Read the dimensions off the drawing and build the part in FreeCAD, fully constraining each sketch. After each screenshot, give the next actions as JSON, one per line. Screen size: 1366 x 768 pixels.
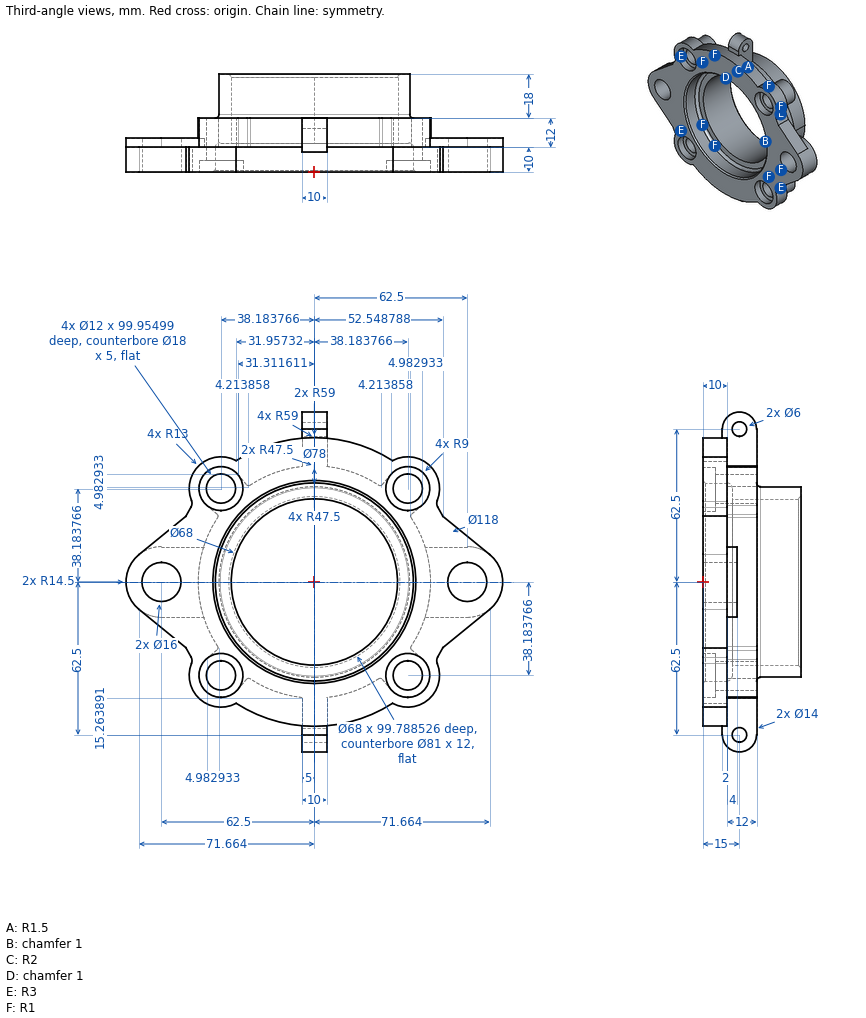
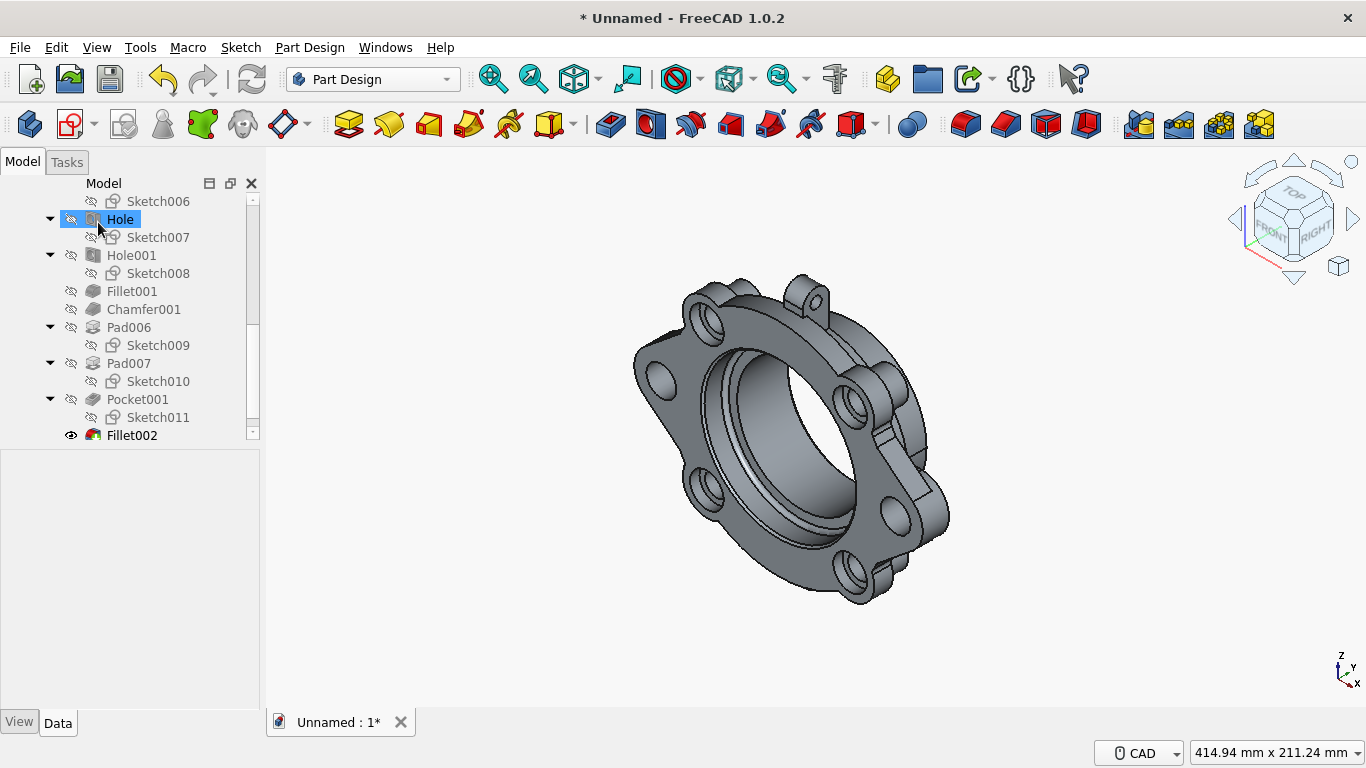
{"action": "key", "text": "2"}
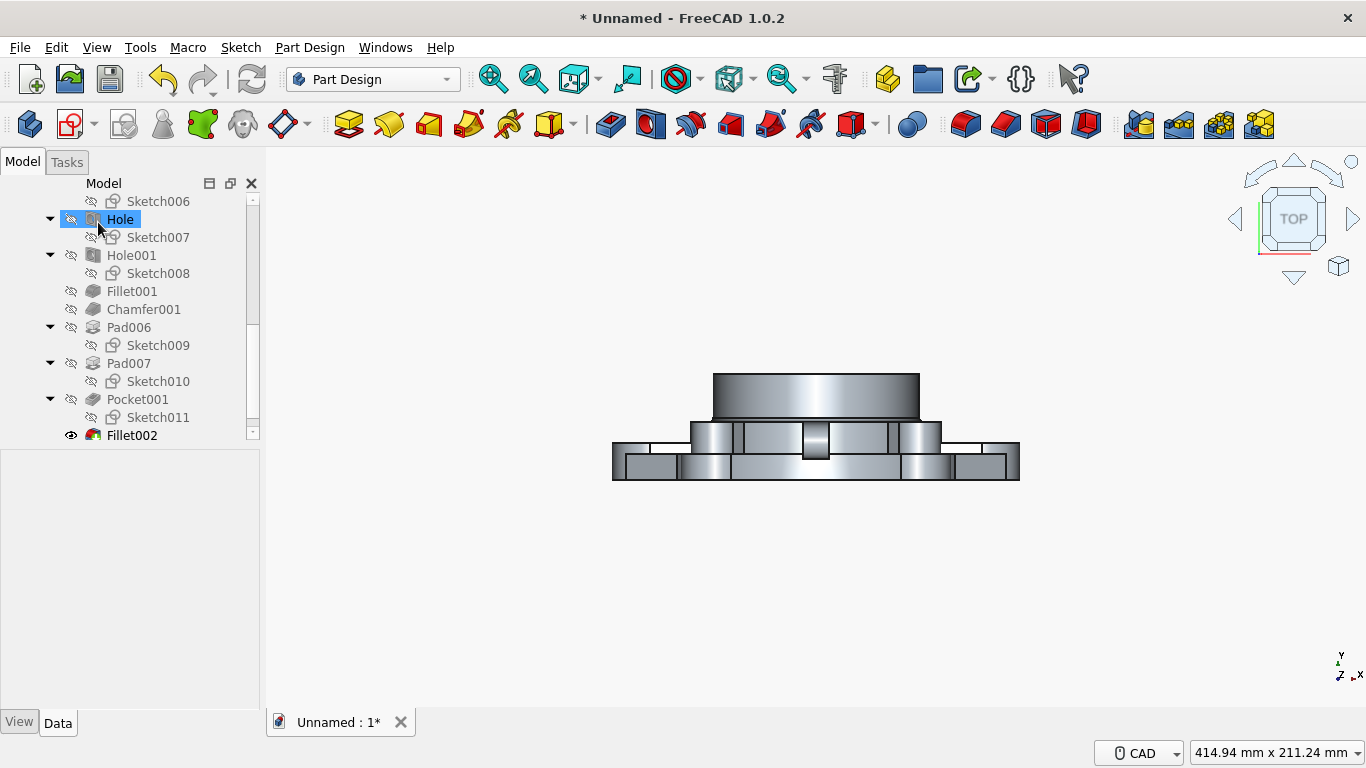
{"action": "left_click", "coordinate": [494, 80]}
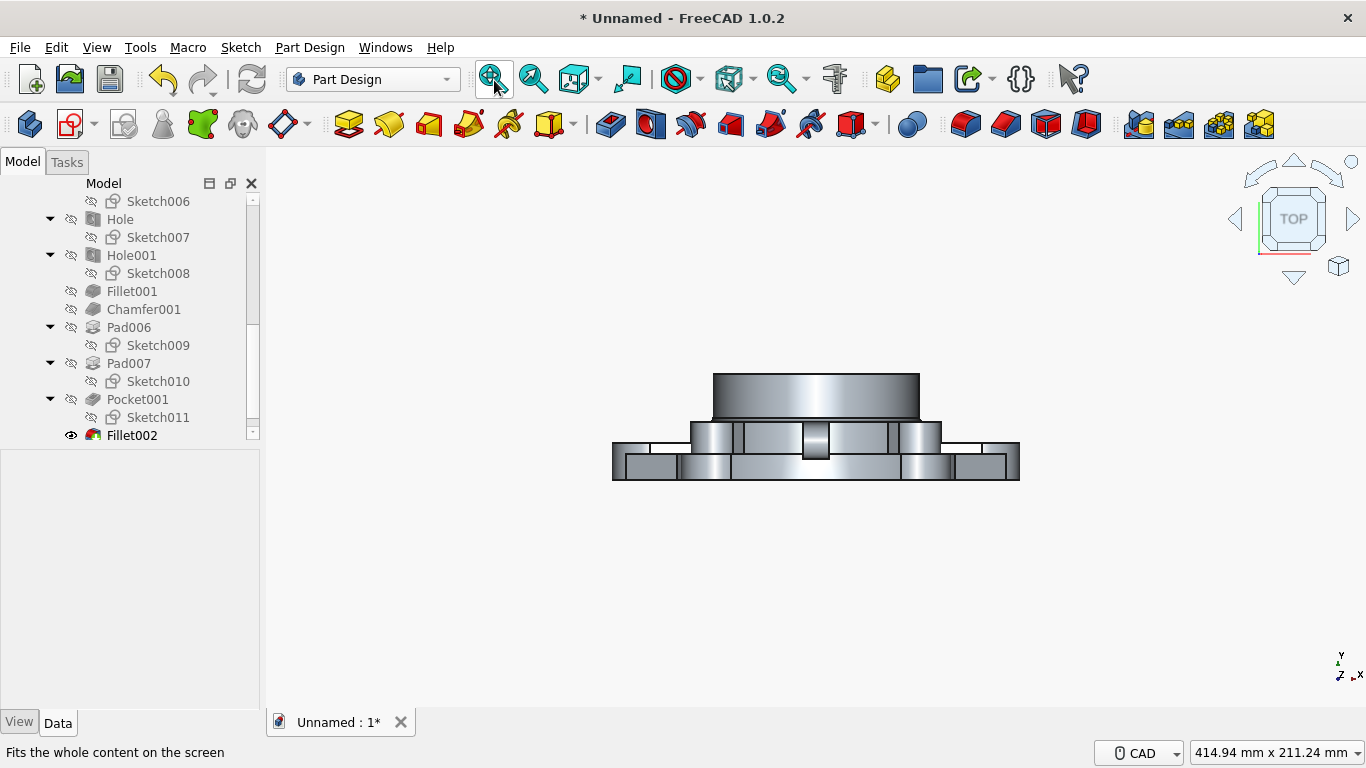
{"action": "key", "text": "1"}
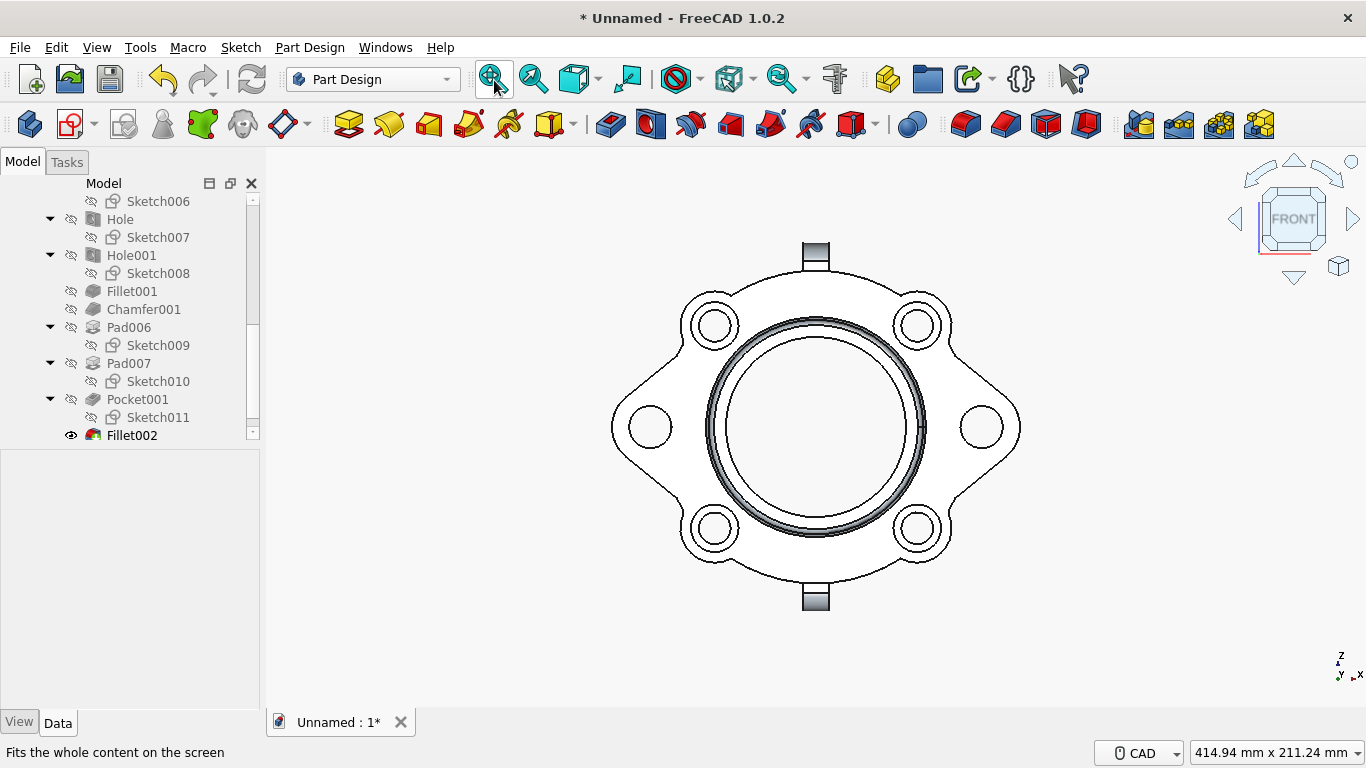
{"action": "key", "text": "3"}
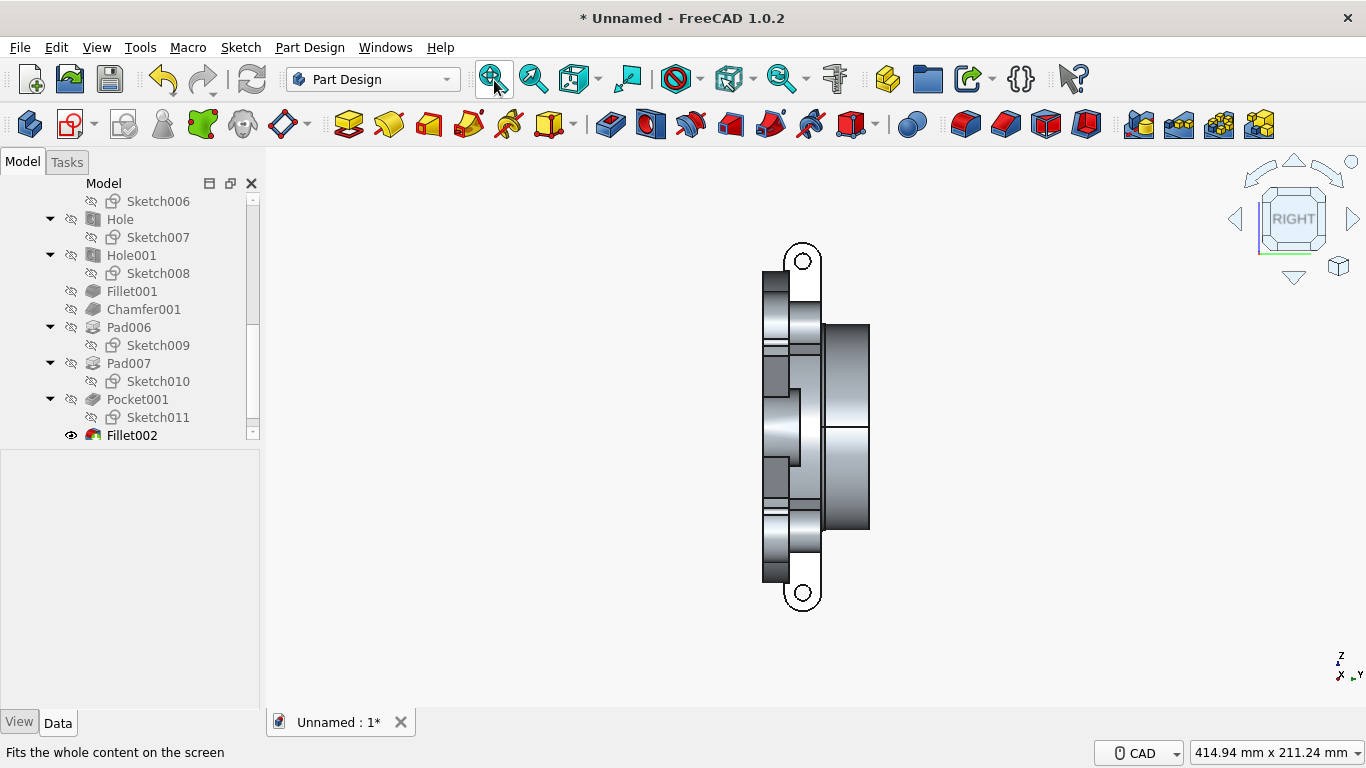
{"action": "key", "text": "5"}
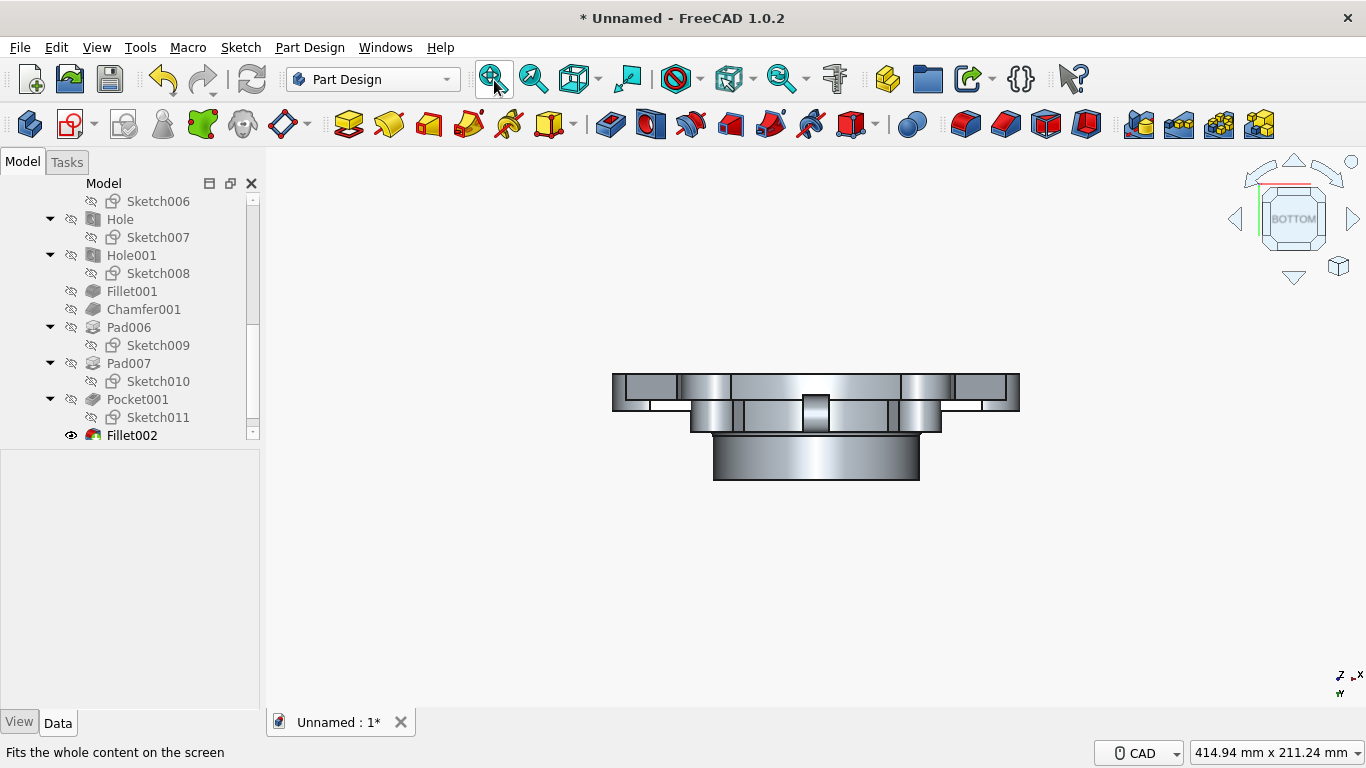
{"action": "left_click", "coordinate": [494, 80]}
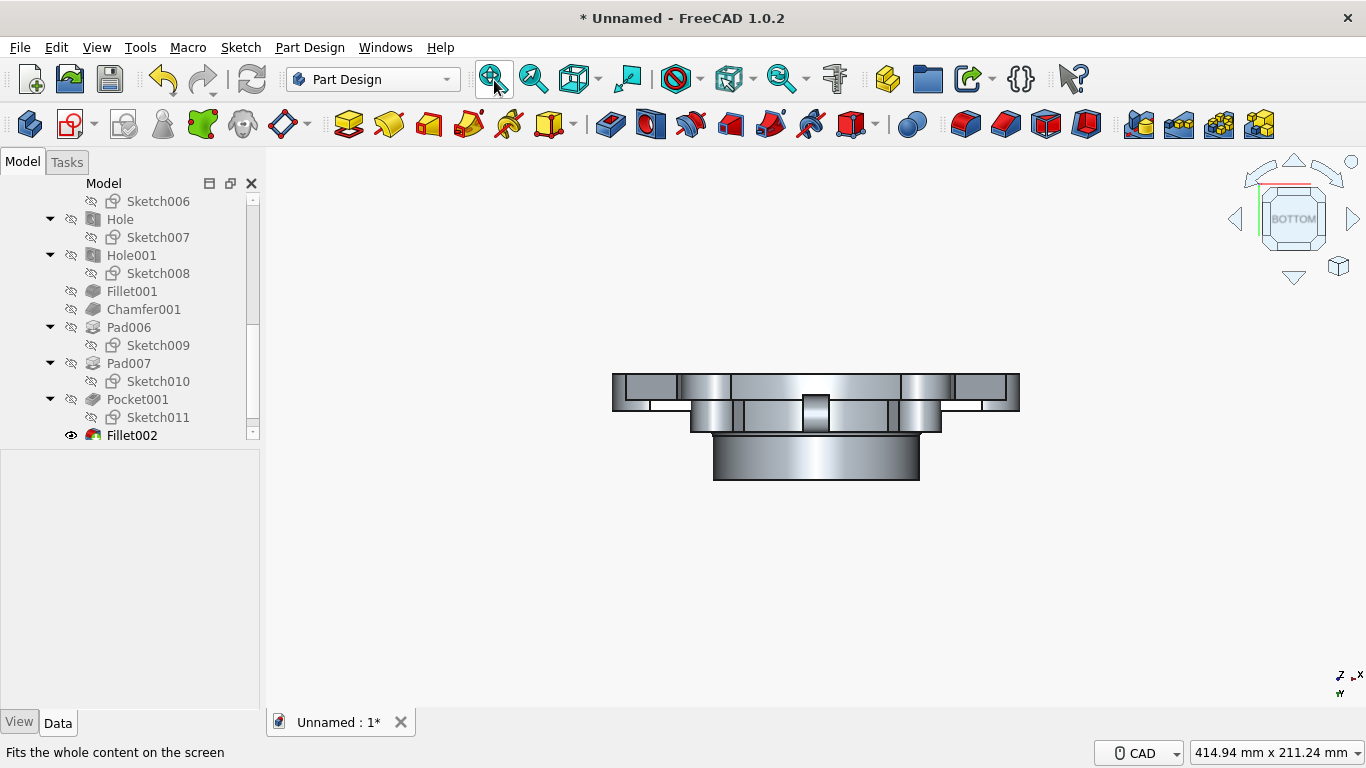
{"action": "key", "text": "4"}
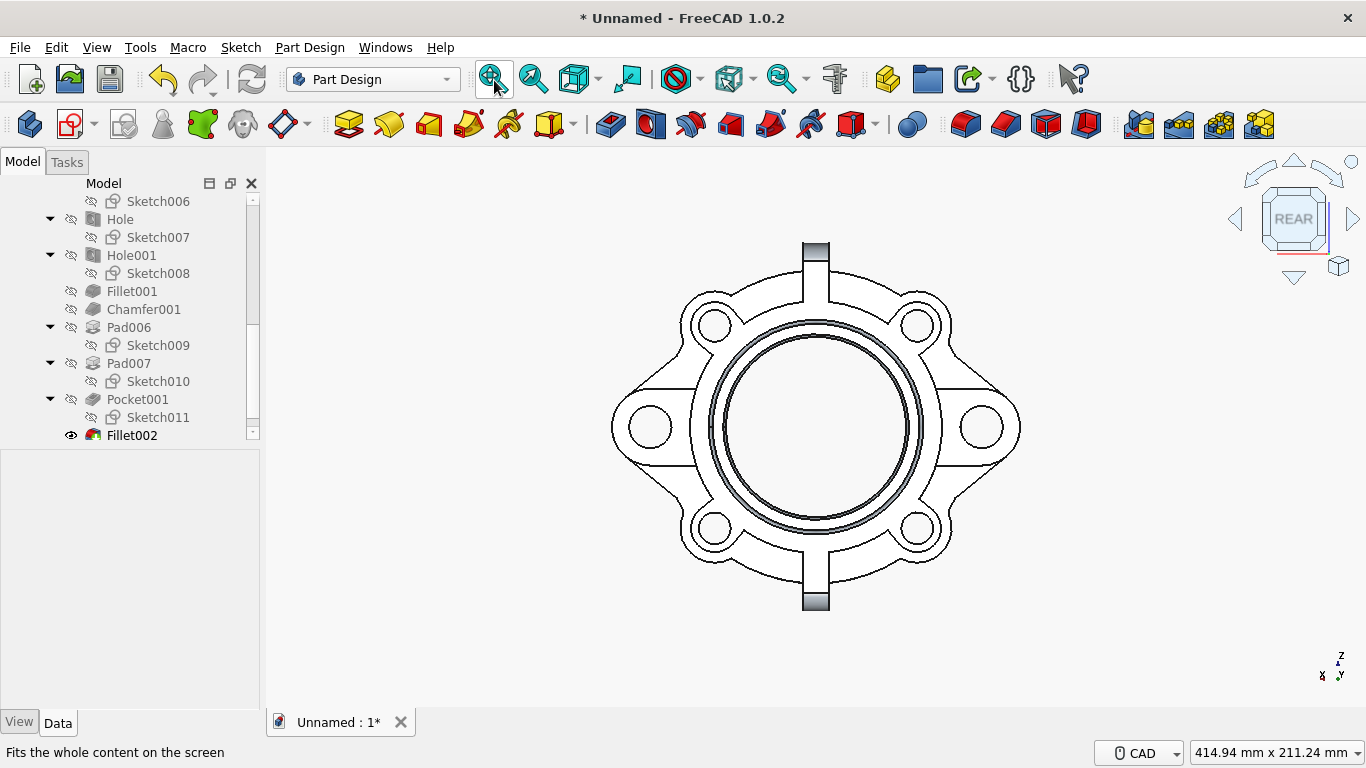
{"action": "key", "text": "6"}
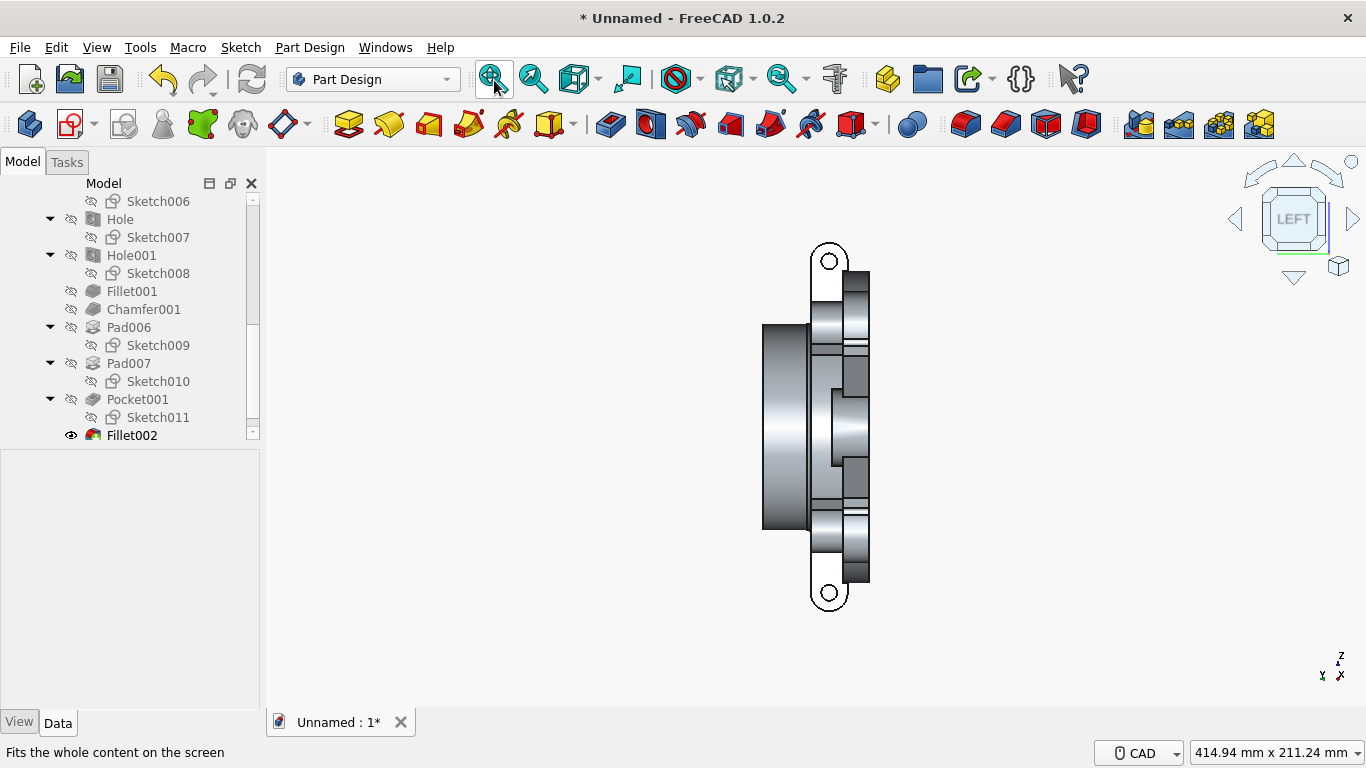
{"action": "key", "text": "v 3"}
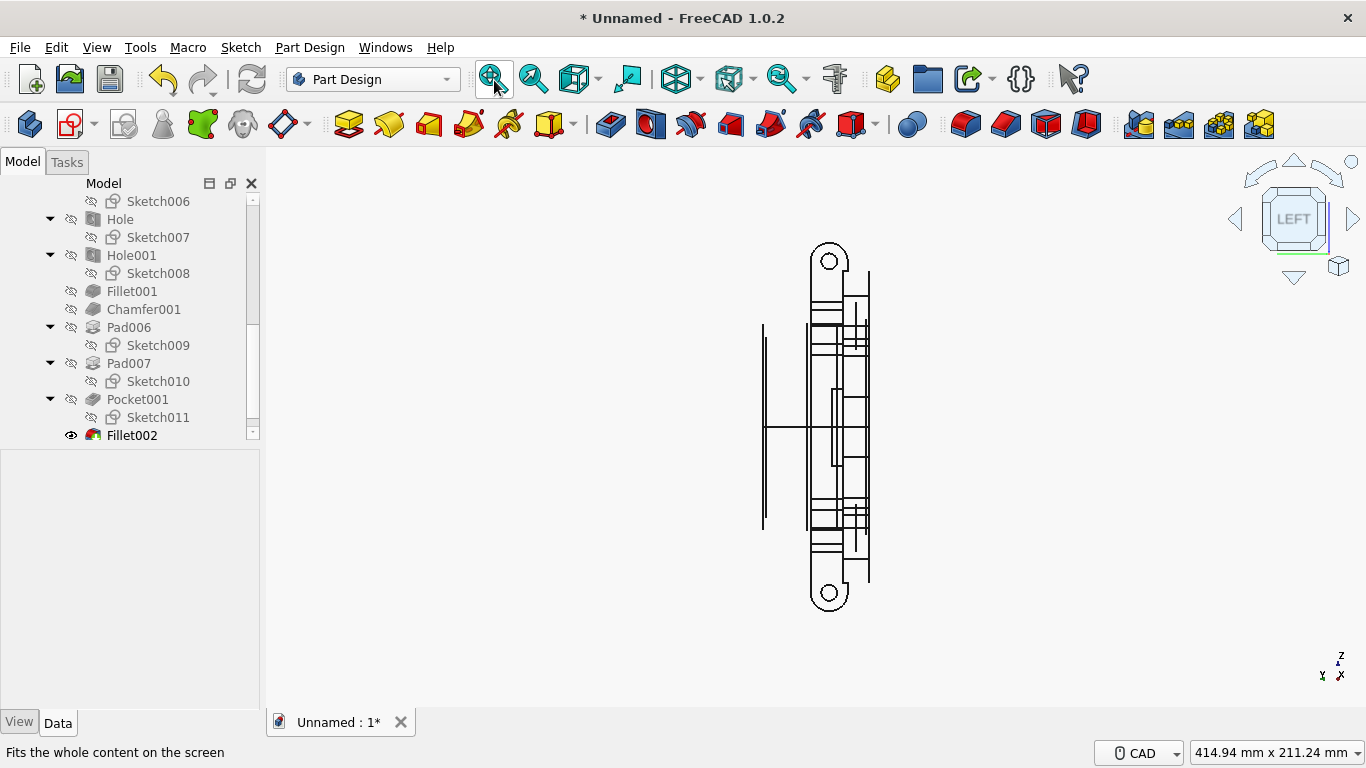
{"action": "key", "text": "0"}